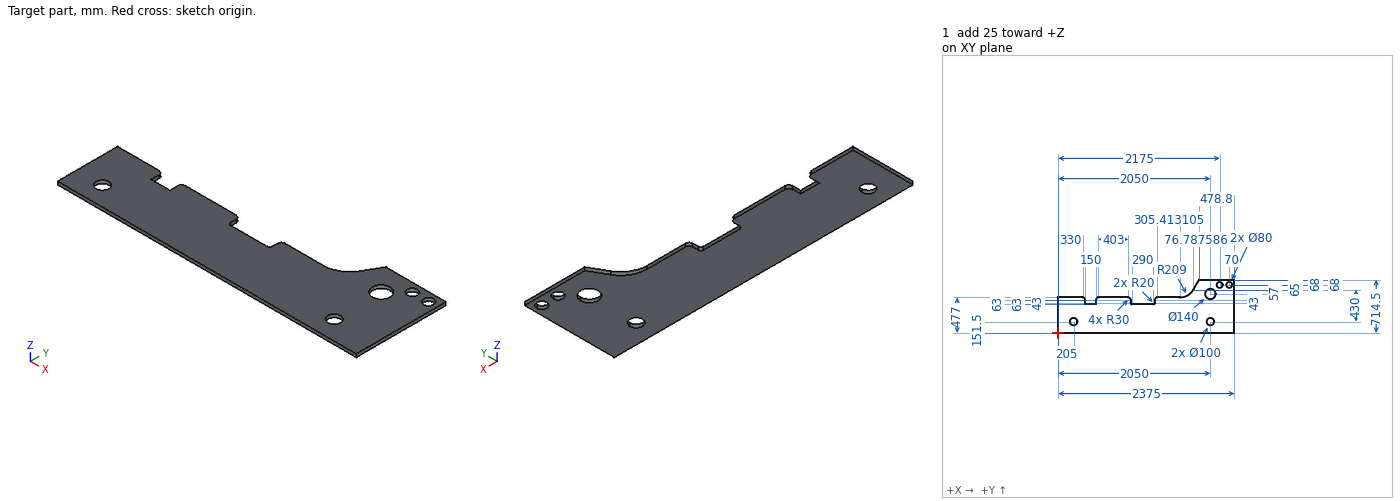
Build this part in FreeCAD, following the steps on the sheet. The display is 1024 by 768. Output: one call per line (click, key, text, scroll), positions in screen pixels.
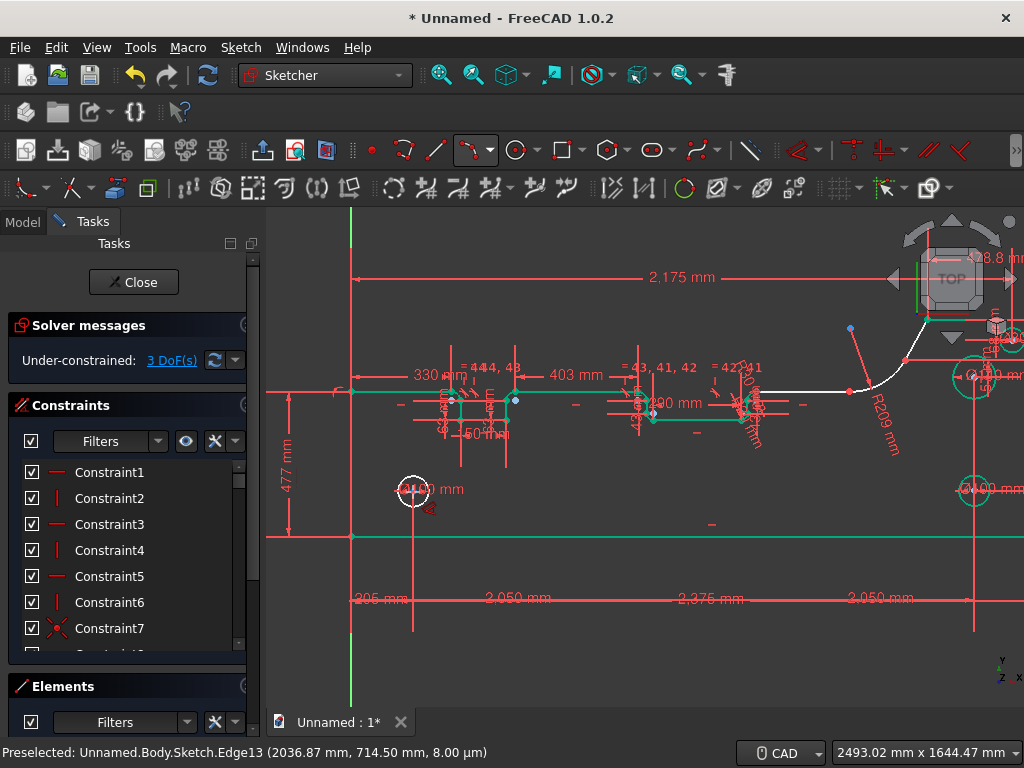
click(413, 491)
click(317, 514)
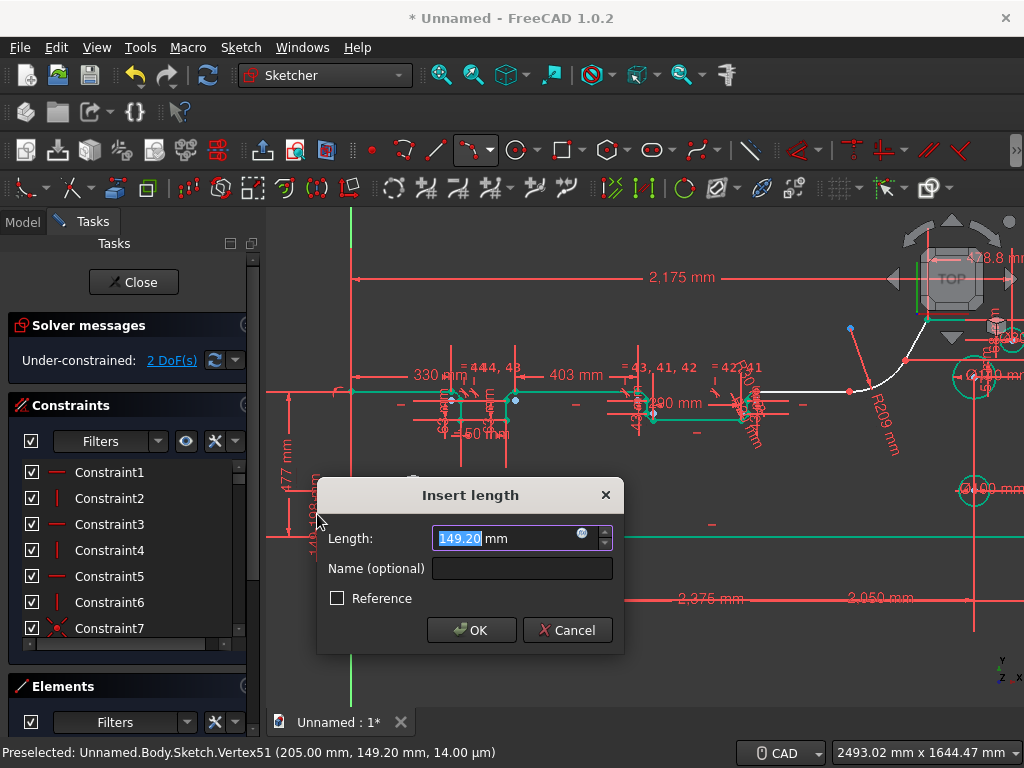
text(151.5)
key(Return)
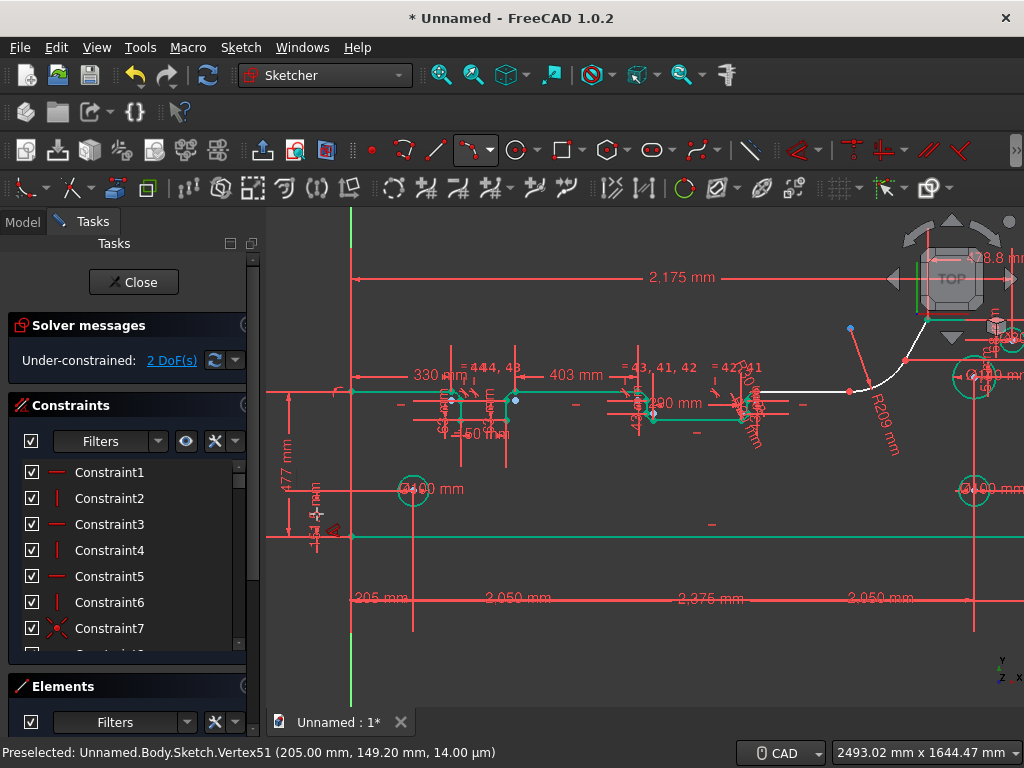
click(822, 392)
click(803, 358)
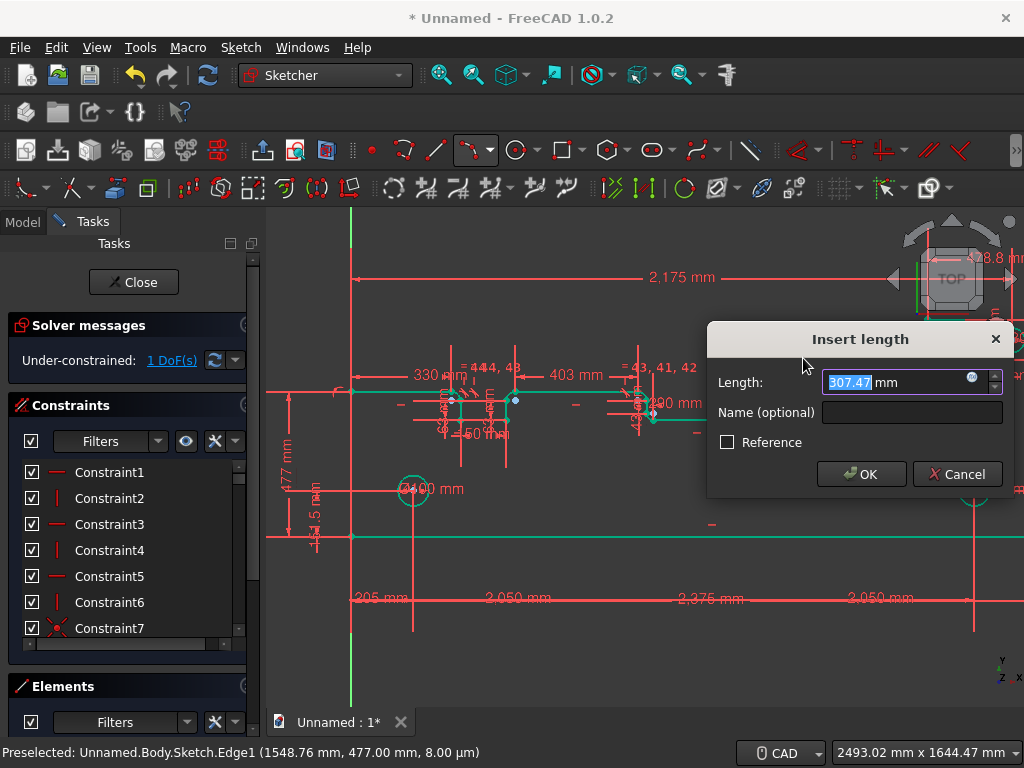
text(305.413105)
key(Return)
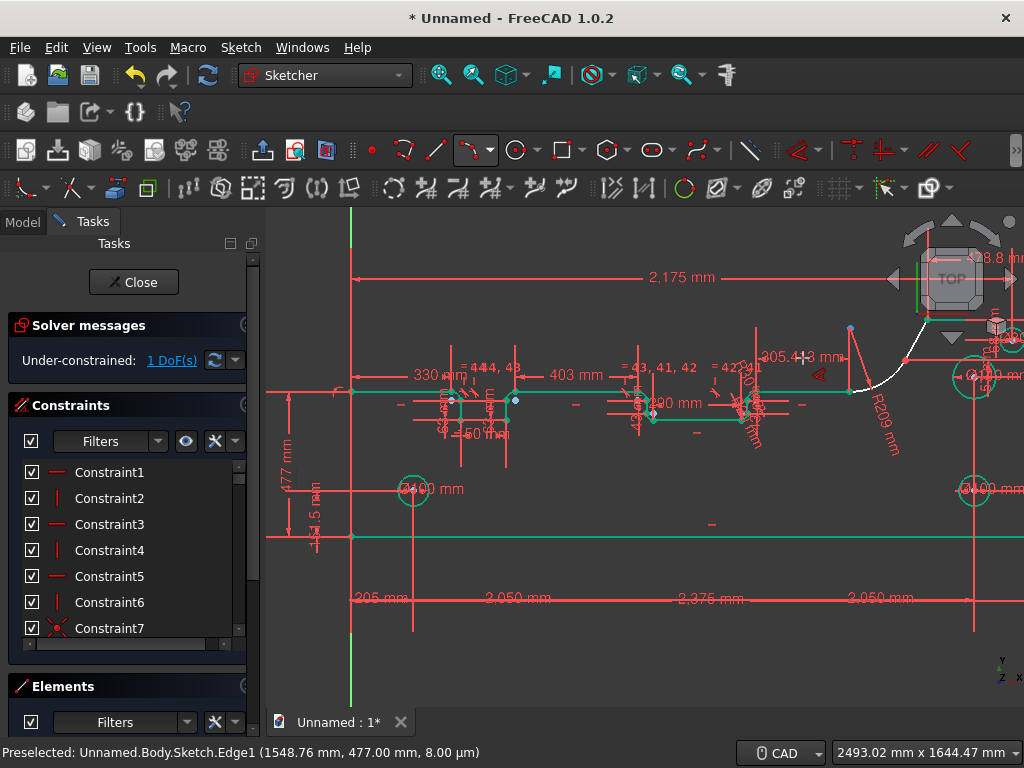
scroll(411, 492, down, 3)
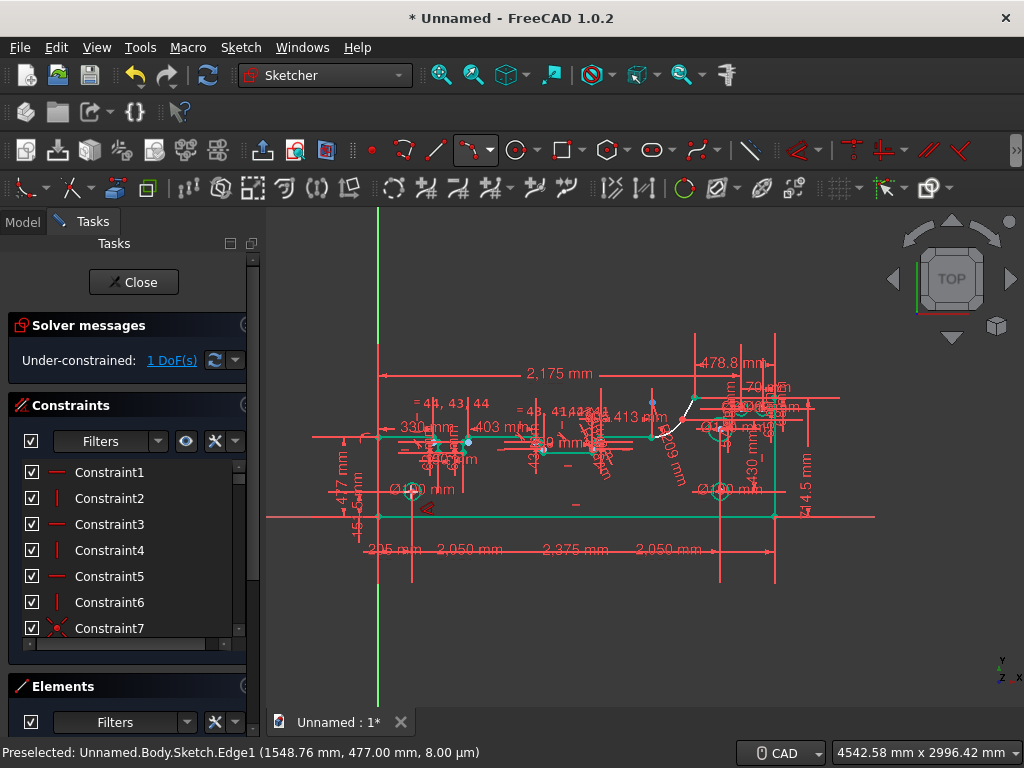
scroll(691, 404, up, 6)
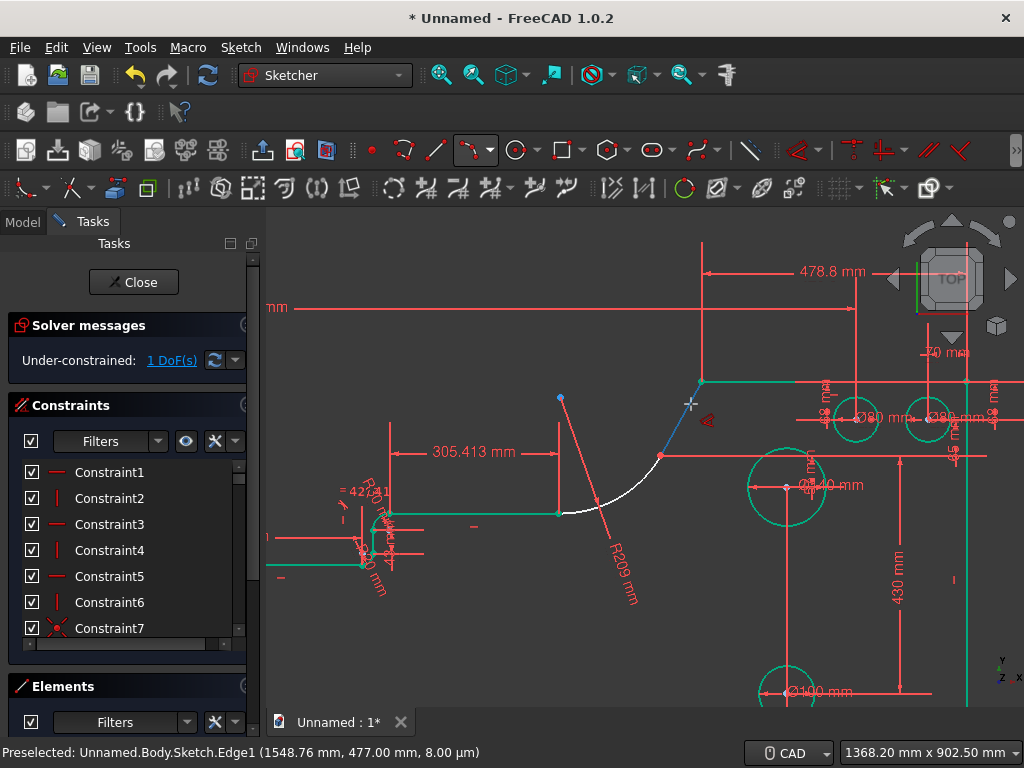
click(689, 404)
click(681, 348)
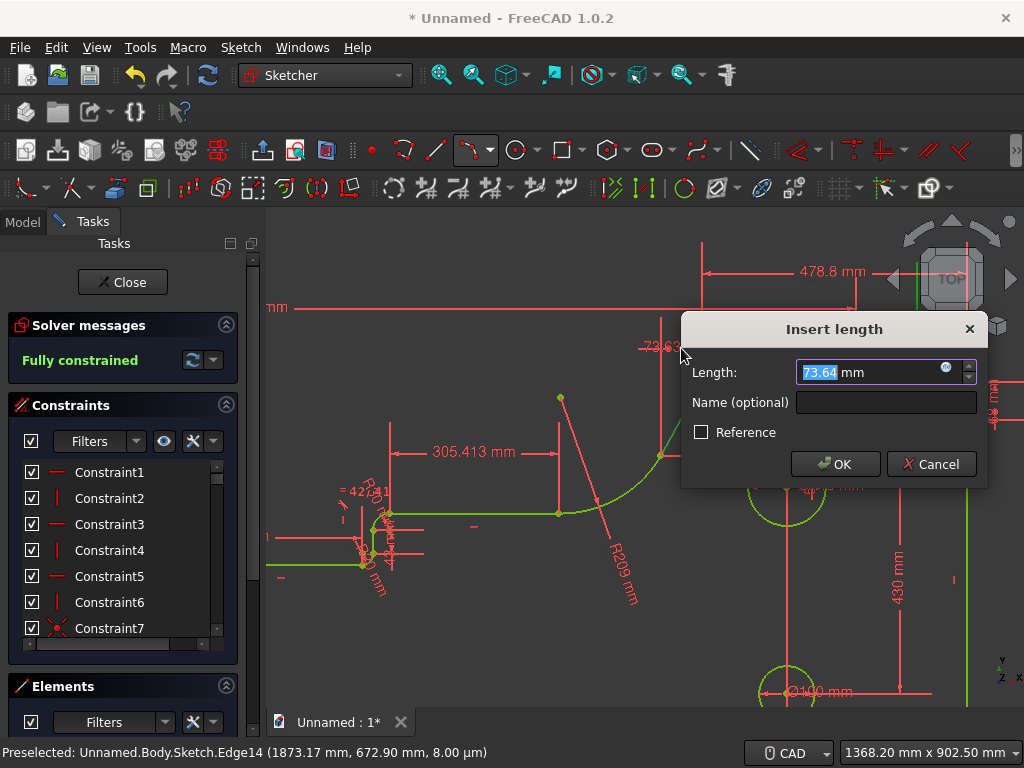
text(76.787586)
key(Return)
key(Escape)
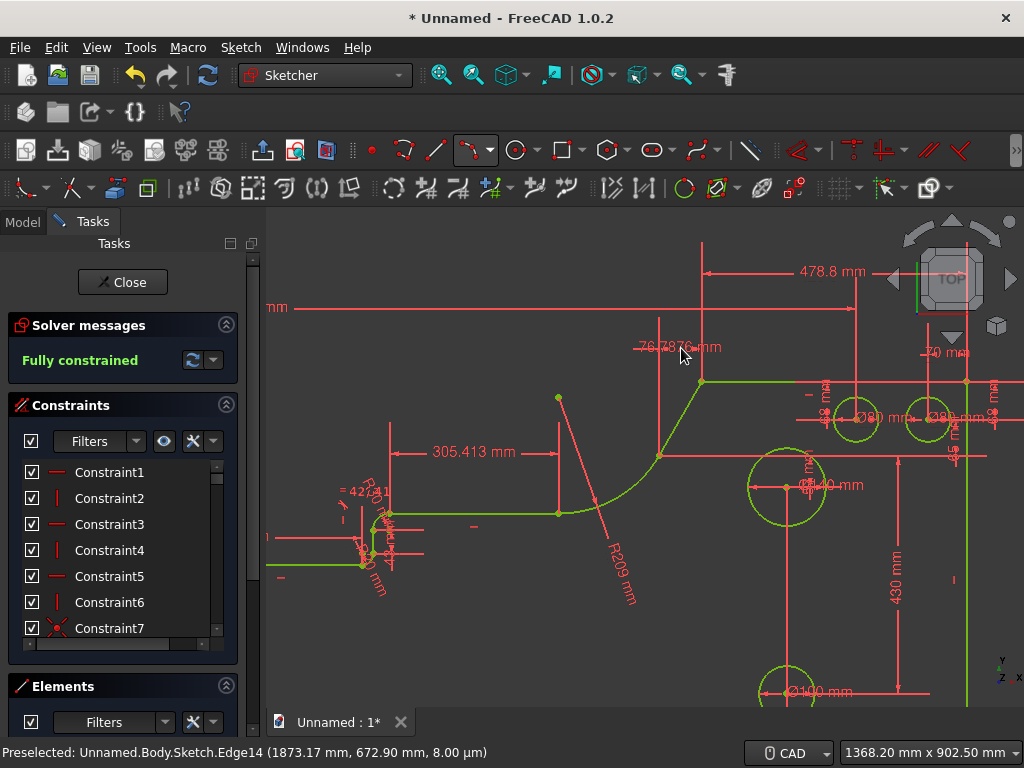
click(123, 282)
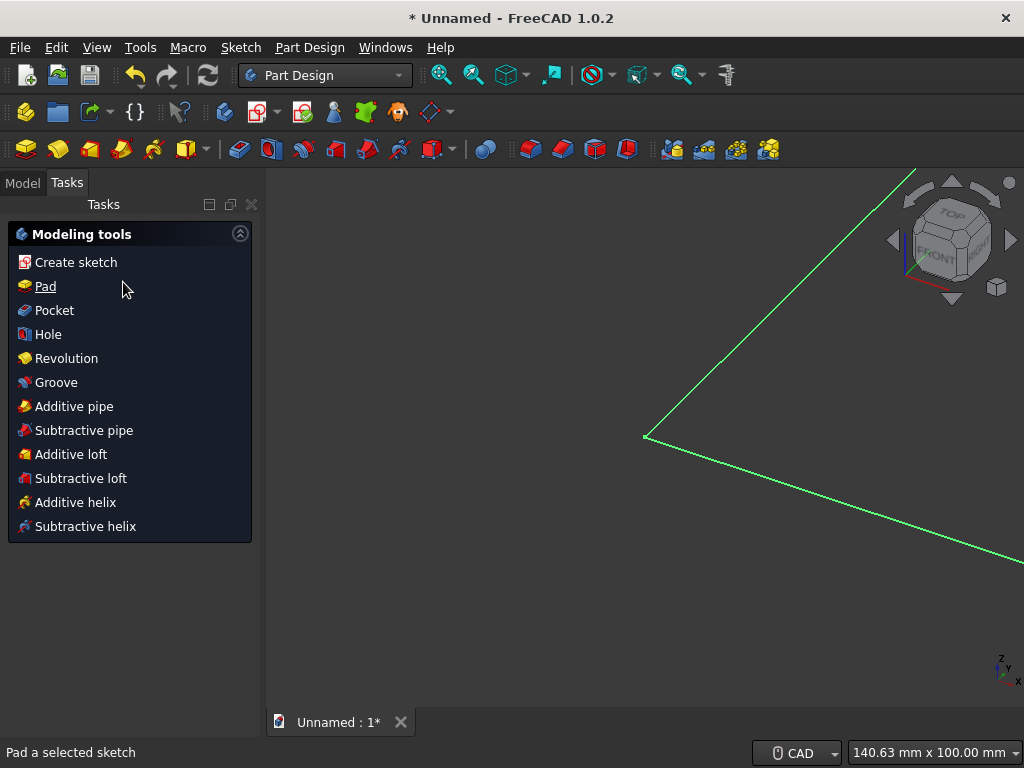
click(26, 150)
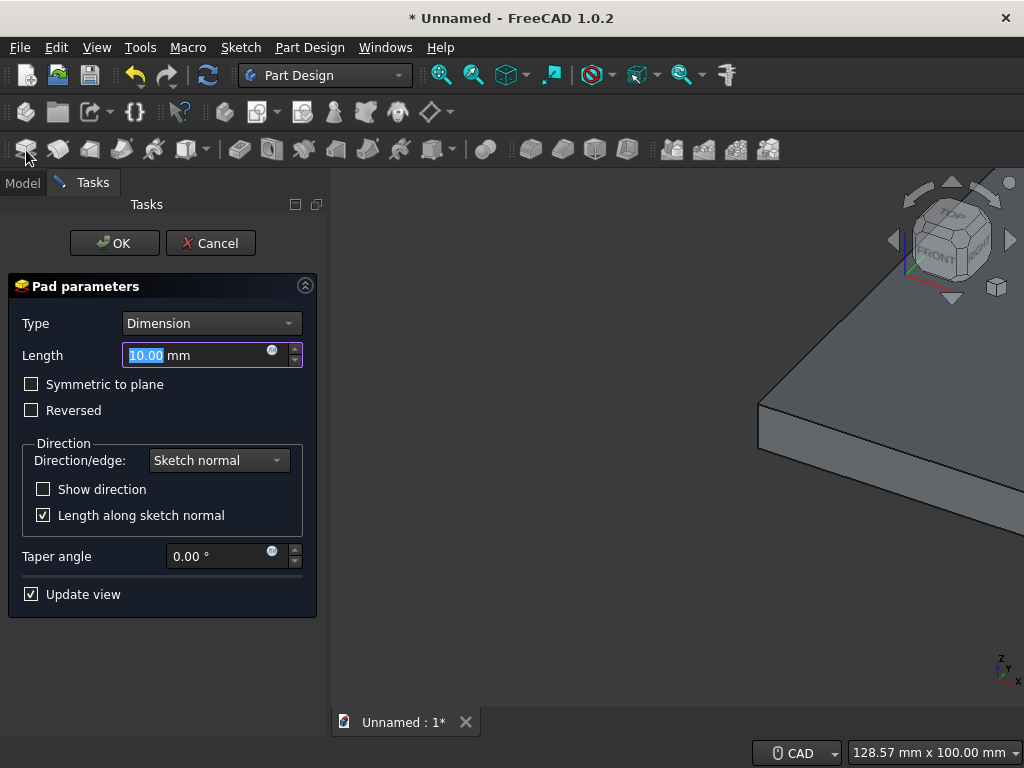
text(25)
key(Tab)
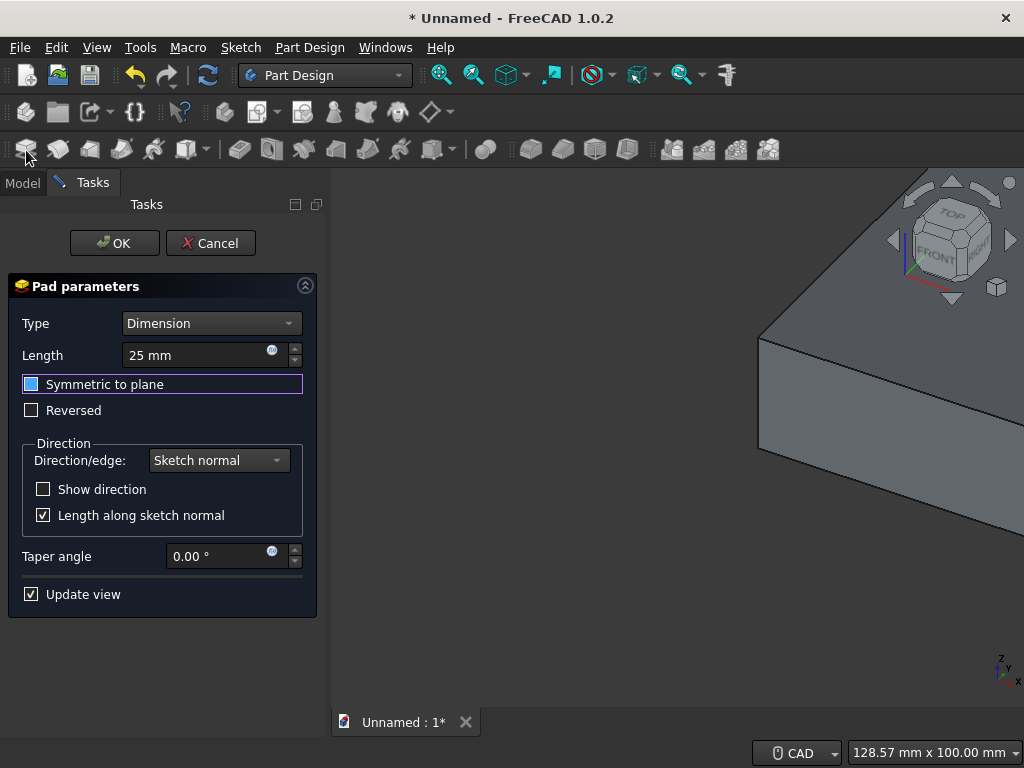
click(115, 243)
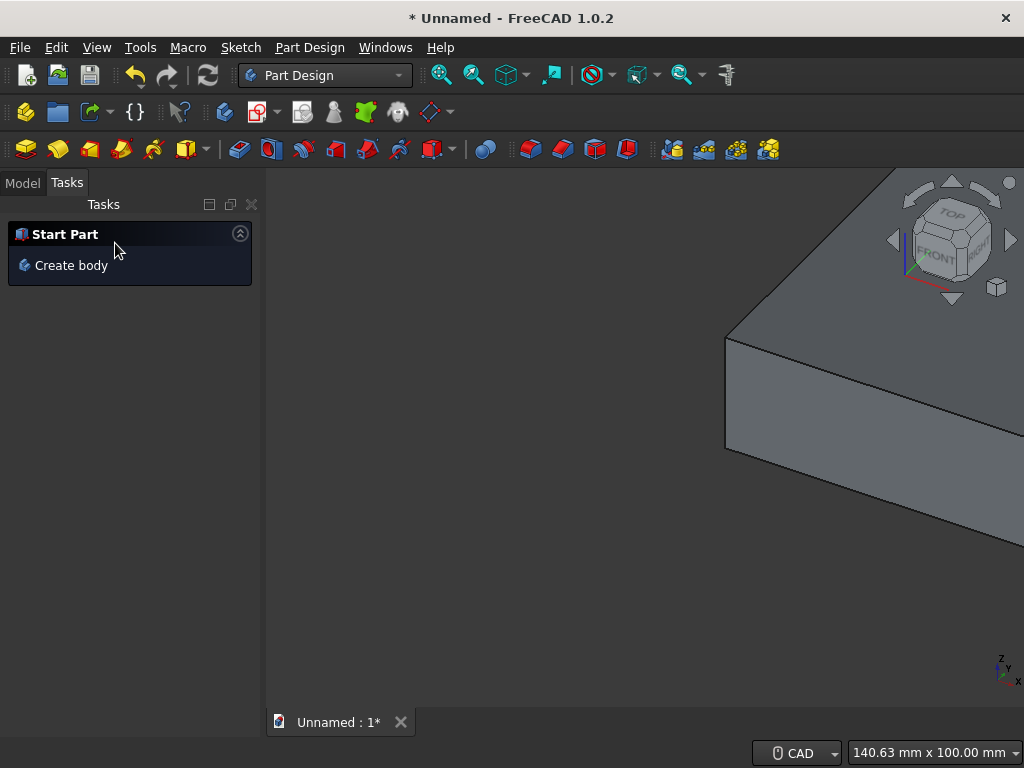
key(0)